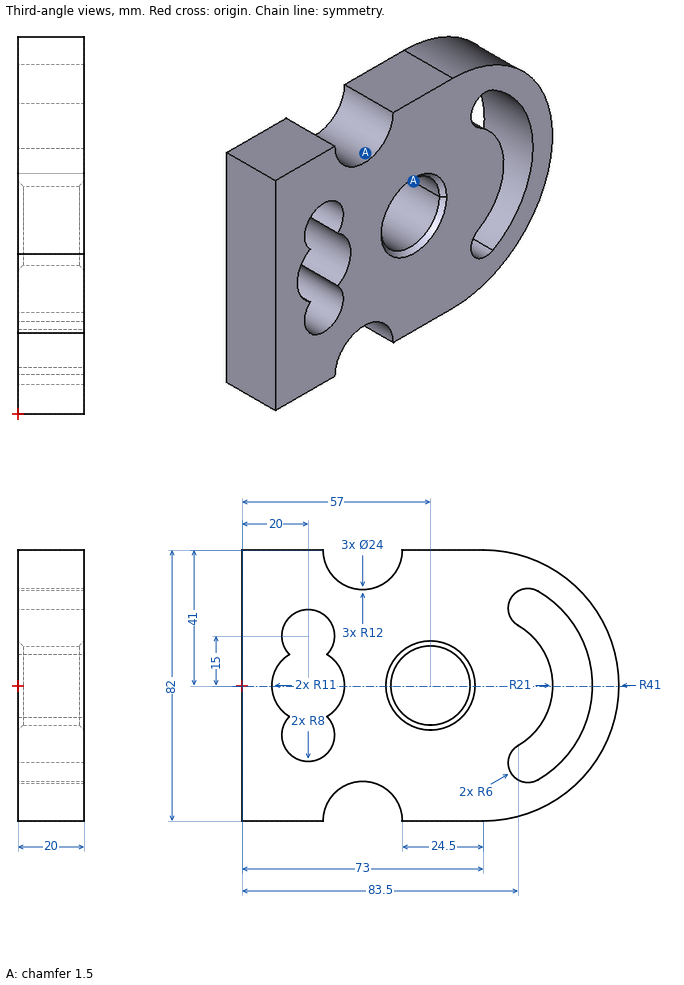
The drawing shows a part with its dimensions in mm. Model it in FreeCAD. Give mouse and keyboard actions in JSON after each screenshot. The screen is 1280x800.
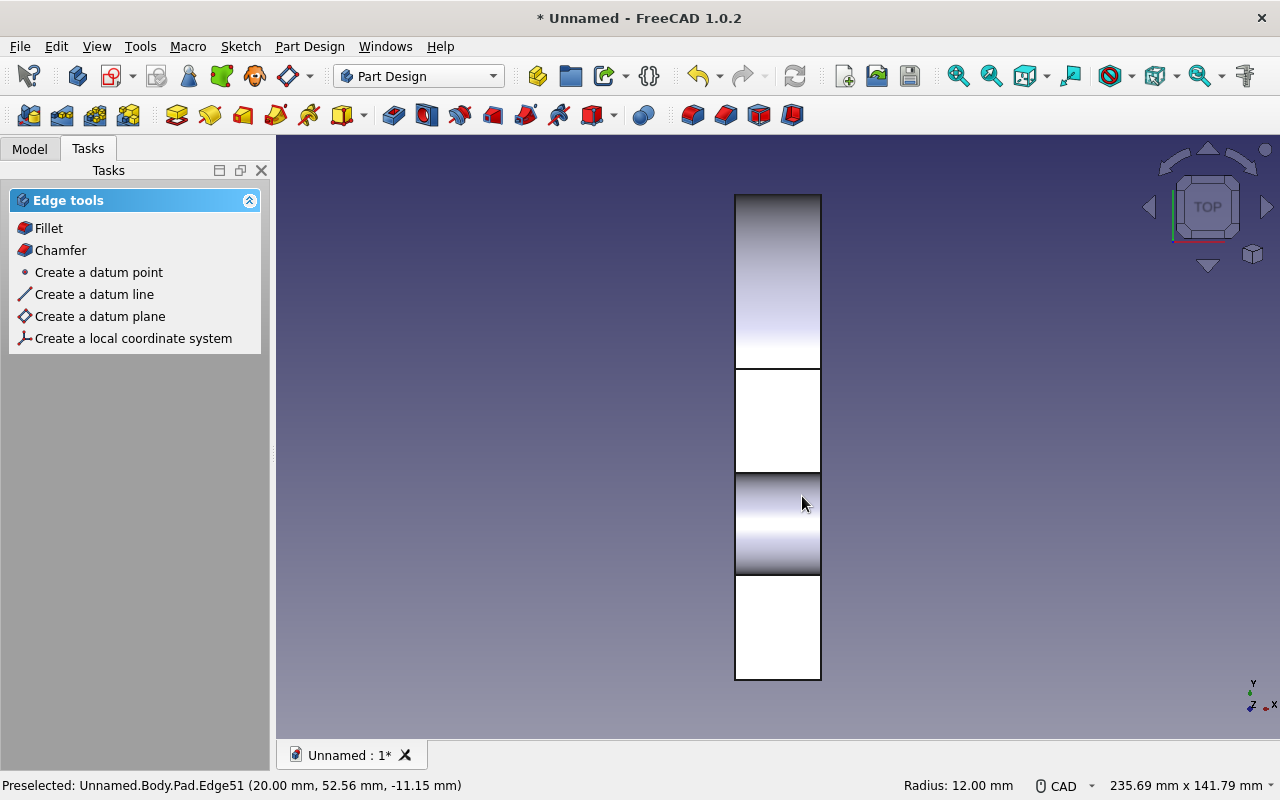
{"action": "key", "text": "1"}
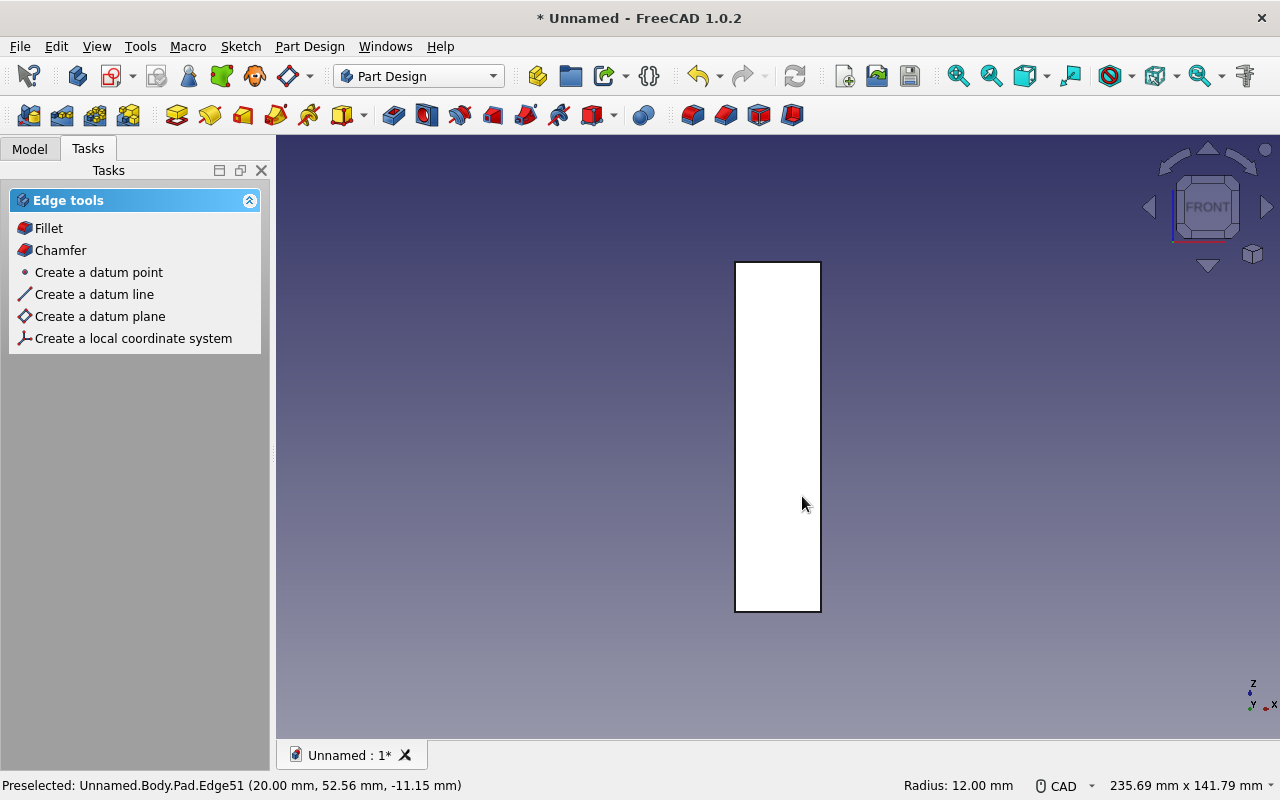
{"action": "key", "text": "3"}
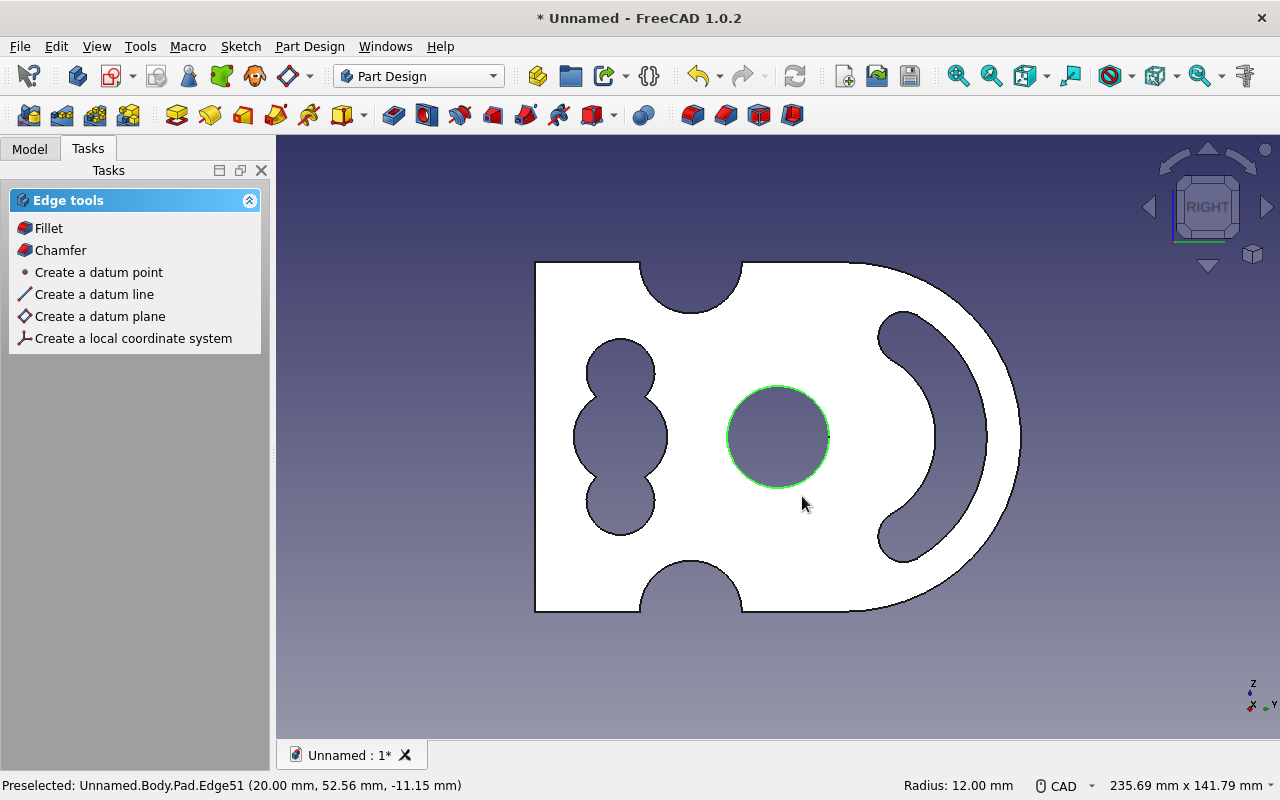
{"action": "key", "text": "5"}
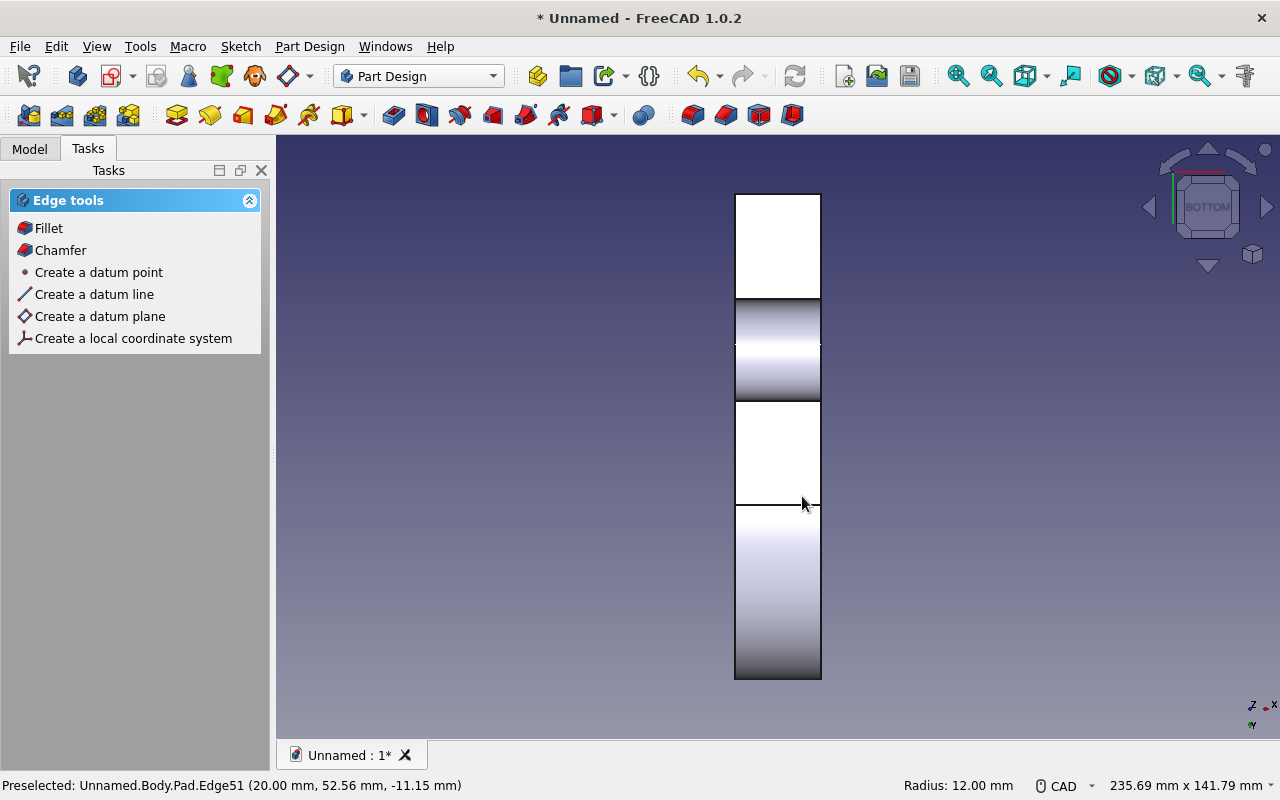
{"action": "key", "text": "4"}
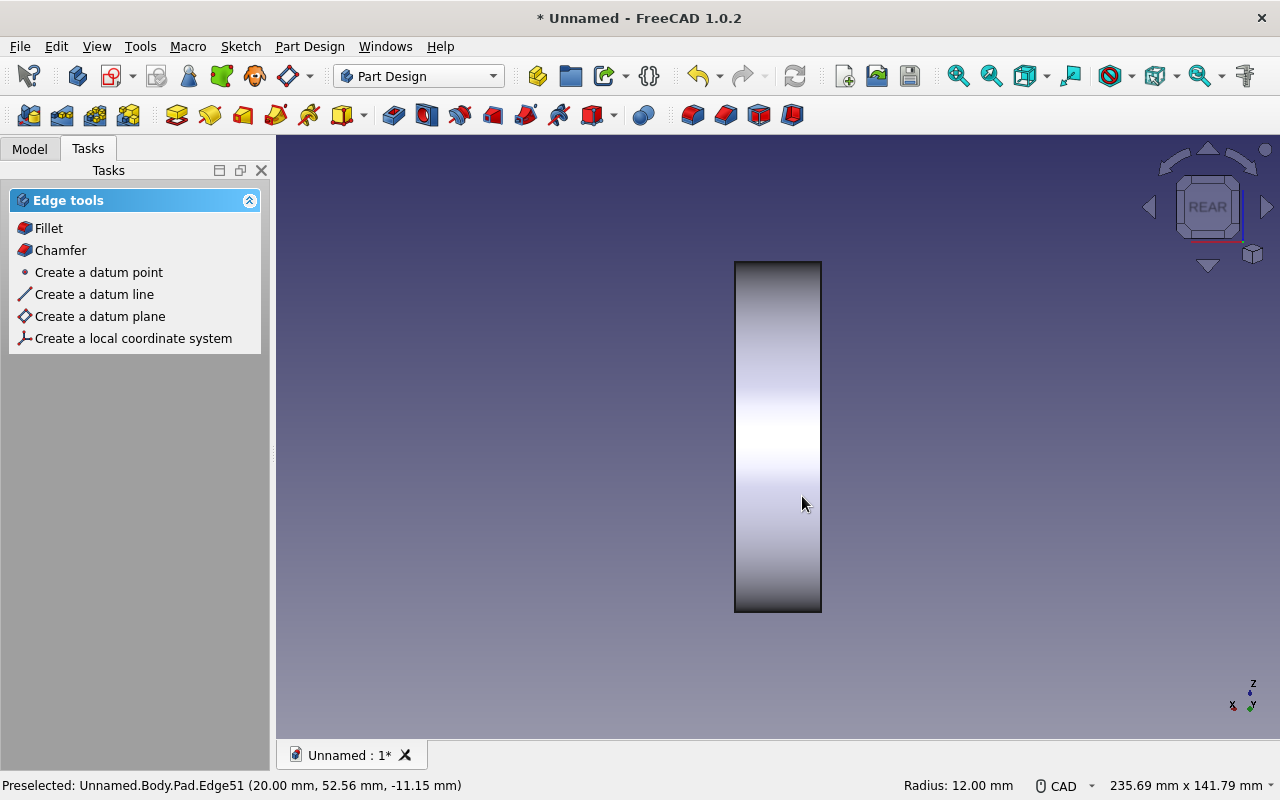
{"action": "key", "text": "6"}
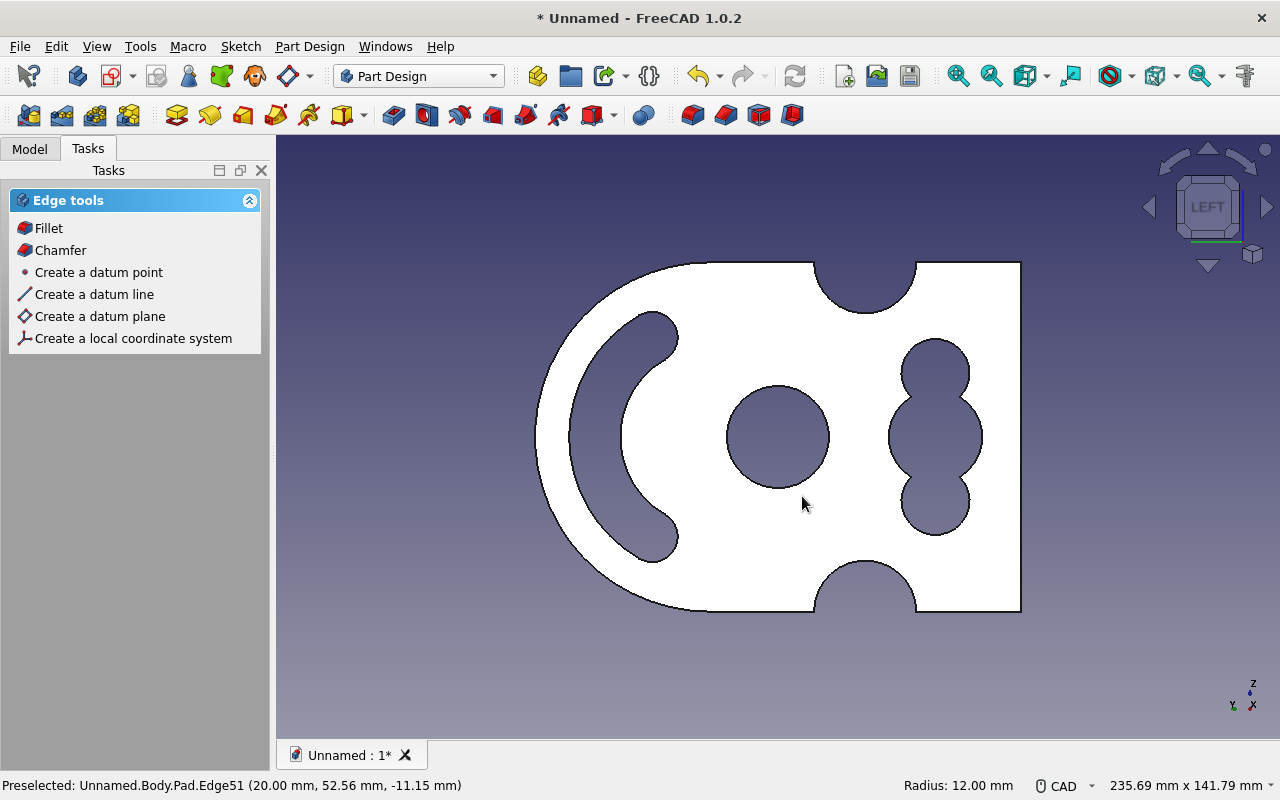
{"action": "key", "text": "v 3"}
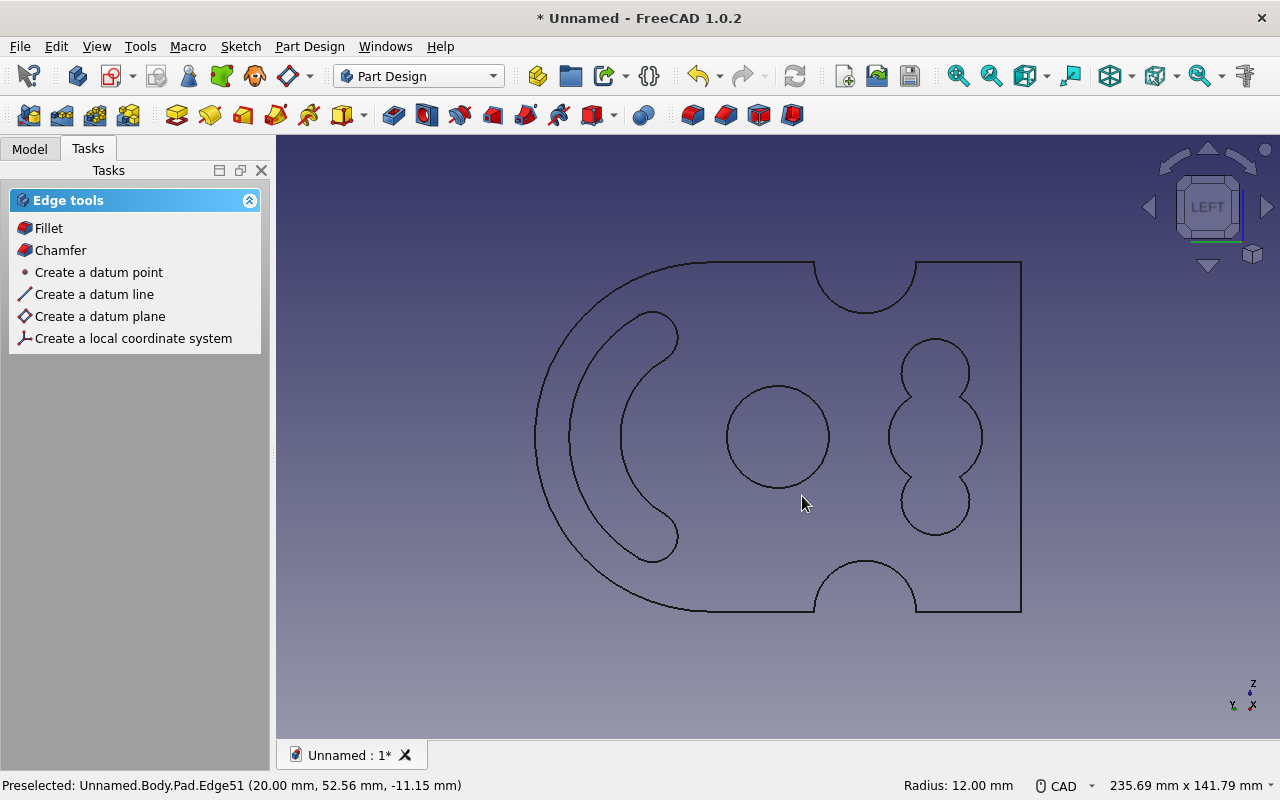
{"action": "key", "text": "0"}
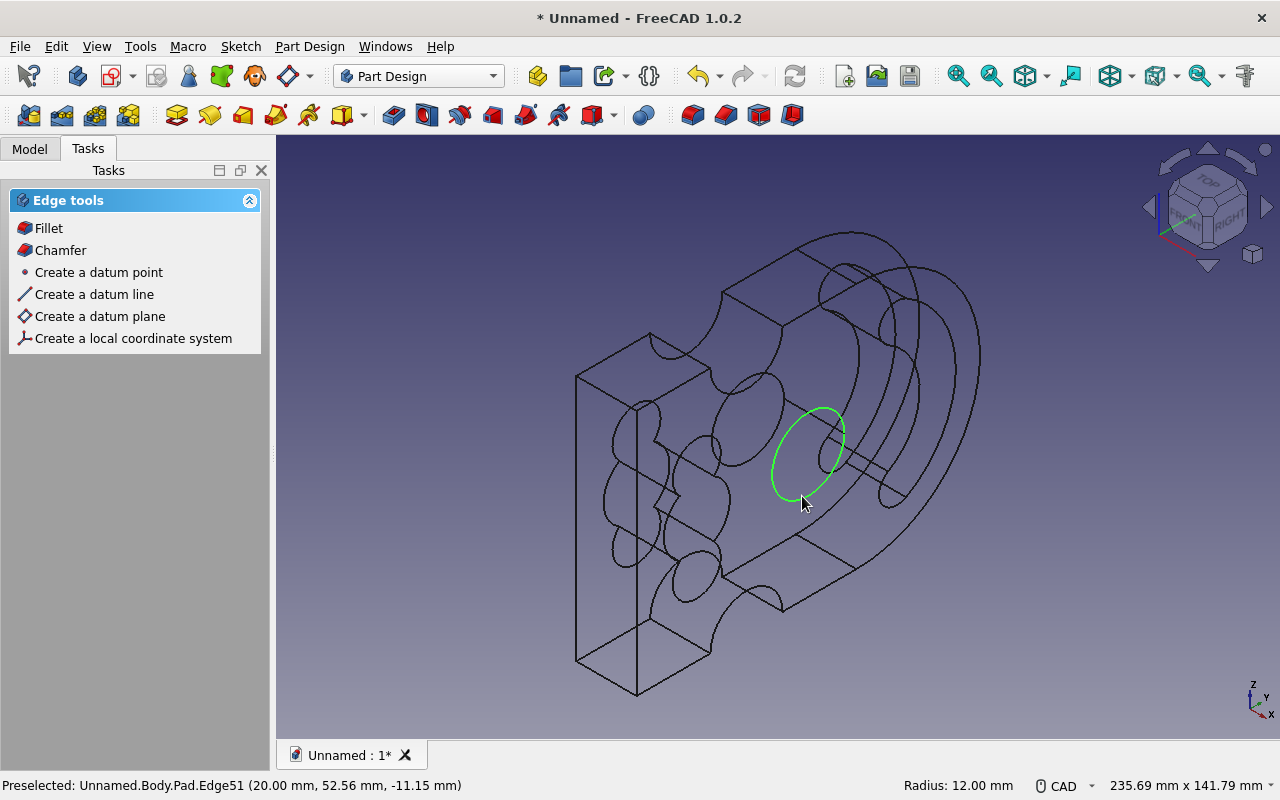
{"action": "left_click", "coordinate": [719, 411], "text": "ctrl"}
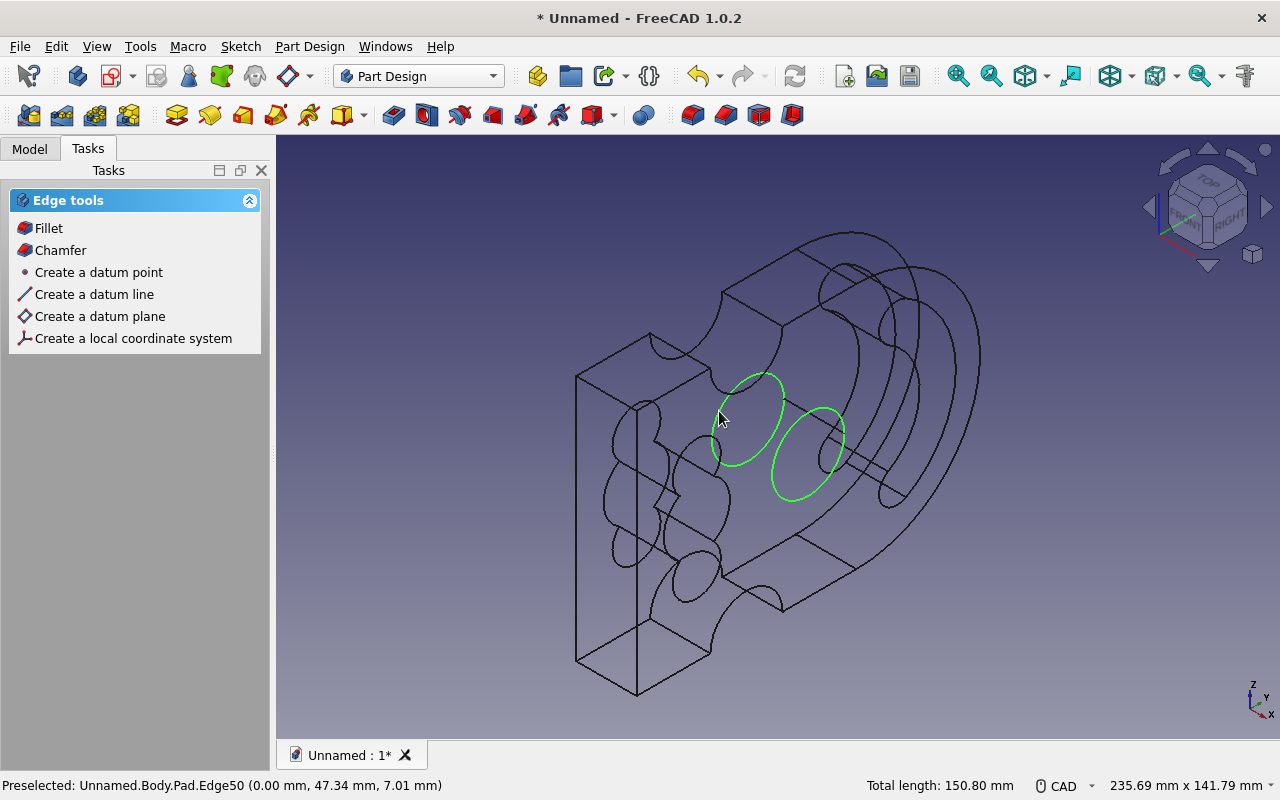
{"action": "key", "text": "v 1"}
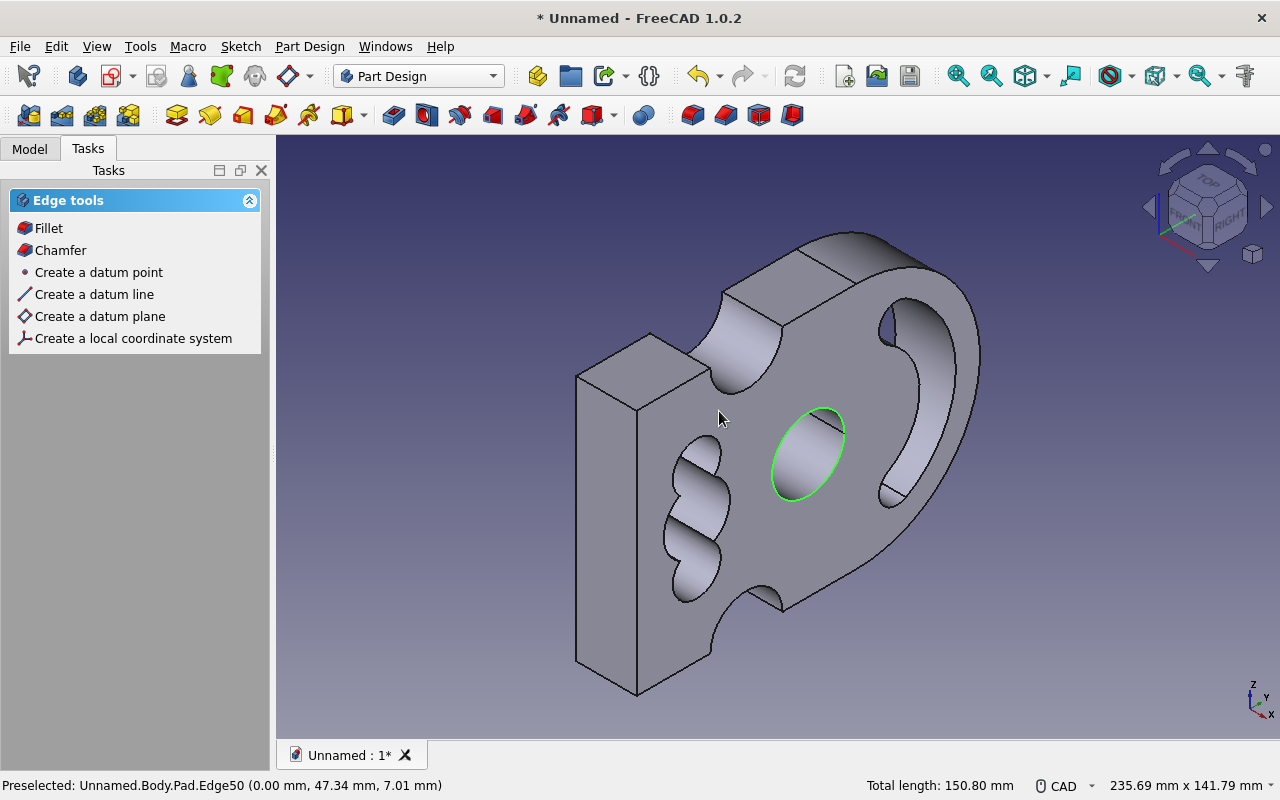
{"action": "left_click", "coordinate": [726, 116]}